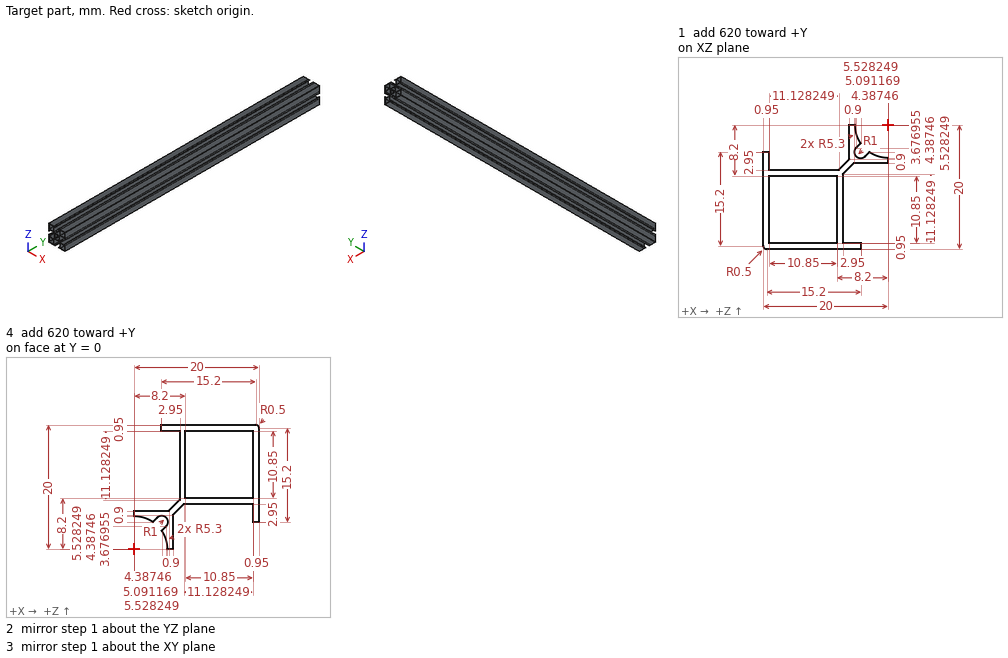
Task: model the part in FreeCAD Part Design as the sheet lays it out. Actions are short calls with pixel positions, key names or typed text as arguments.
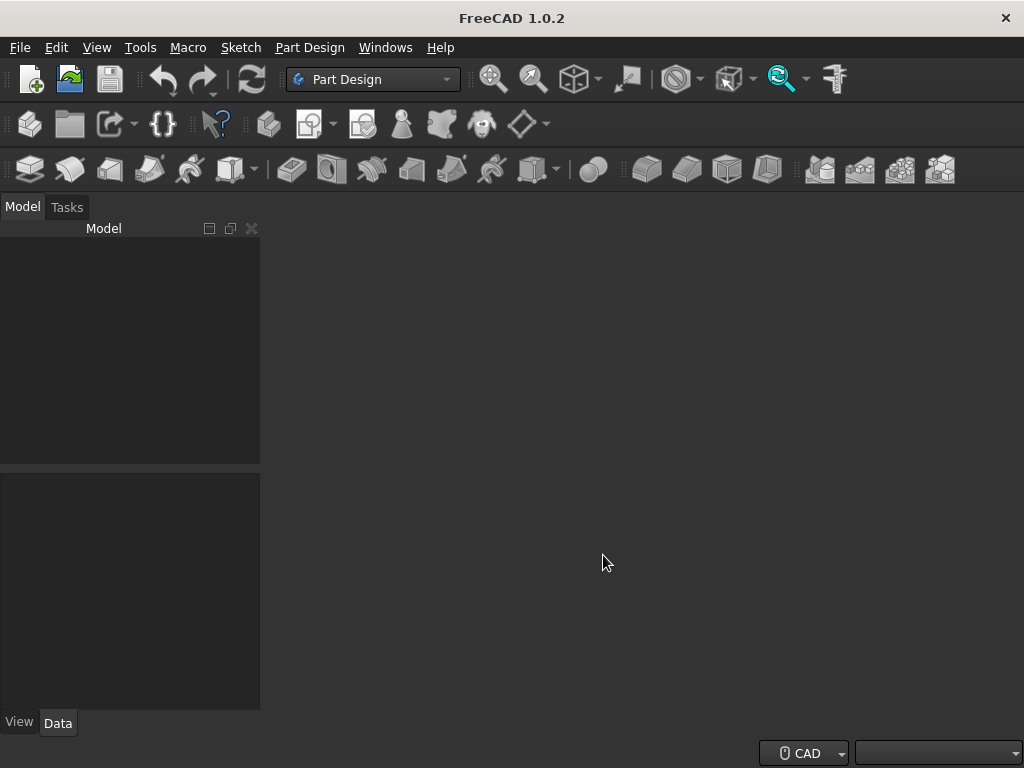
click(30, 80)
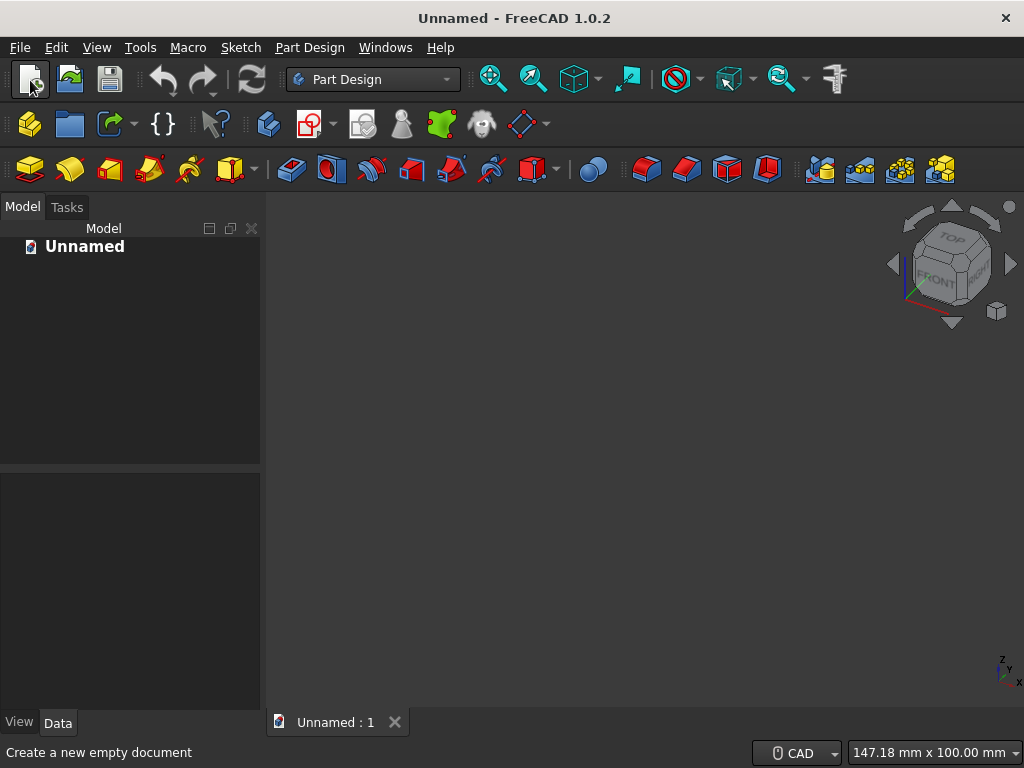
click(310, 124)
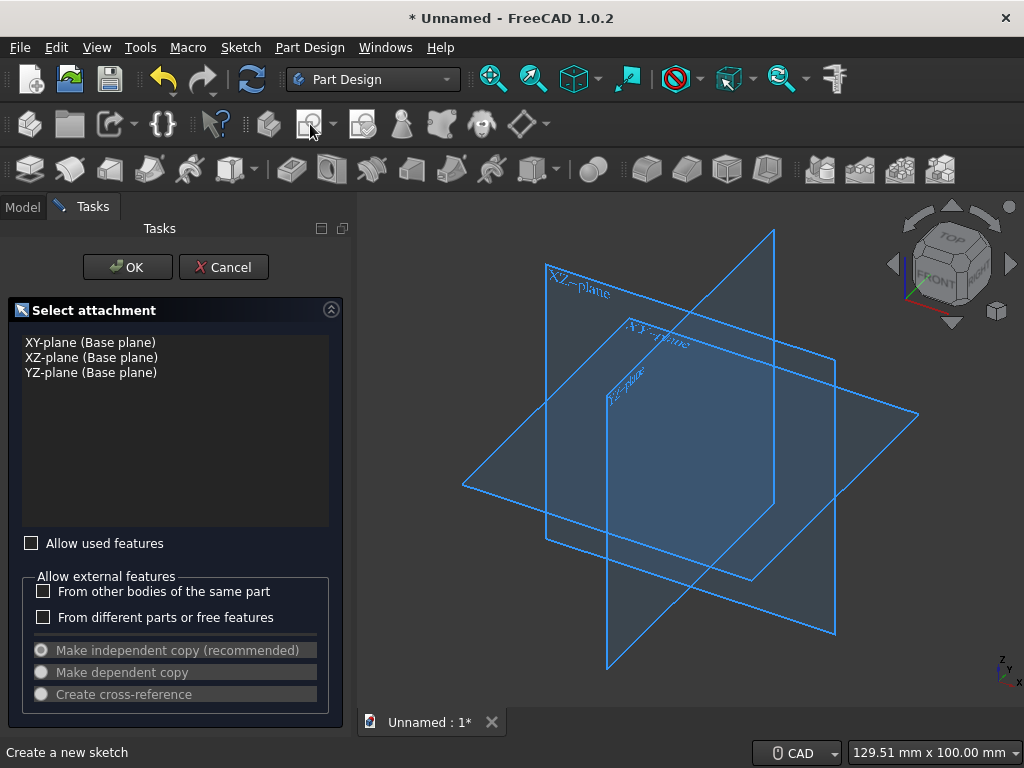
click(82, 358)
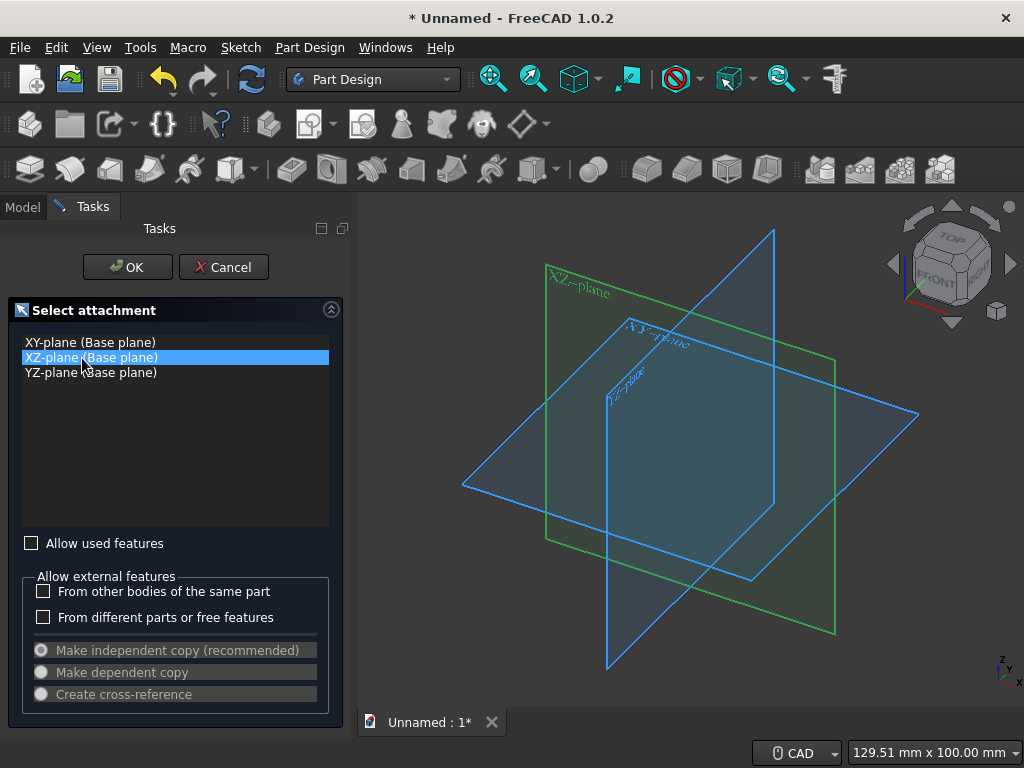
click(128, 267)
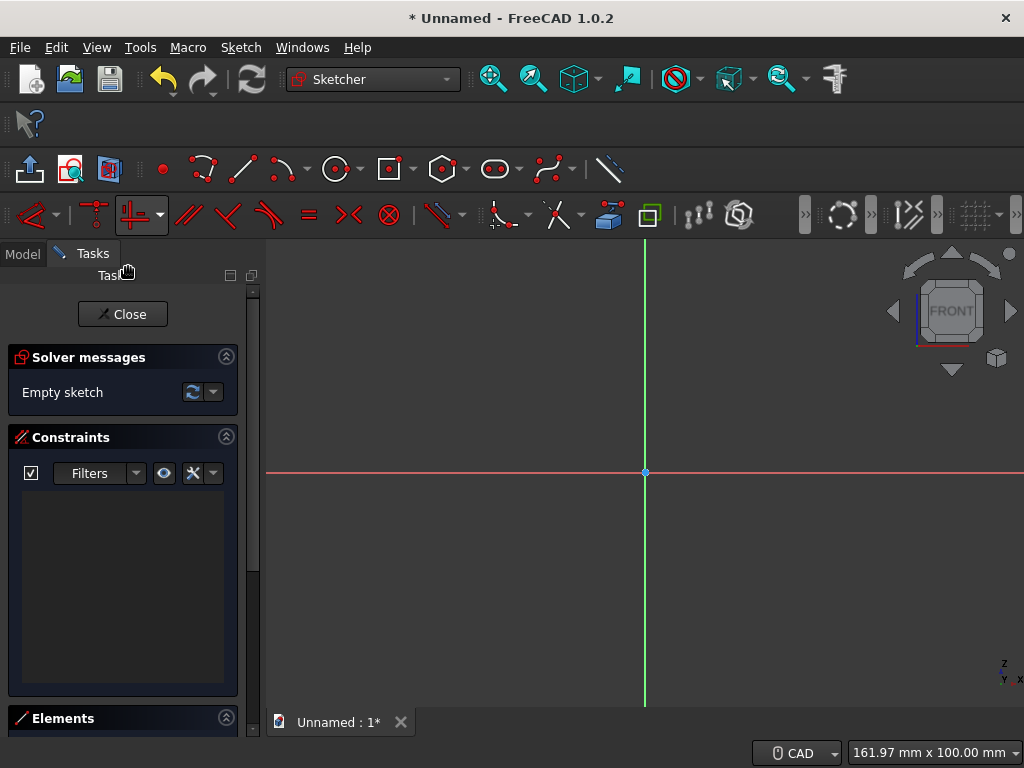
scroll(608, 540, up, 6)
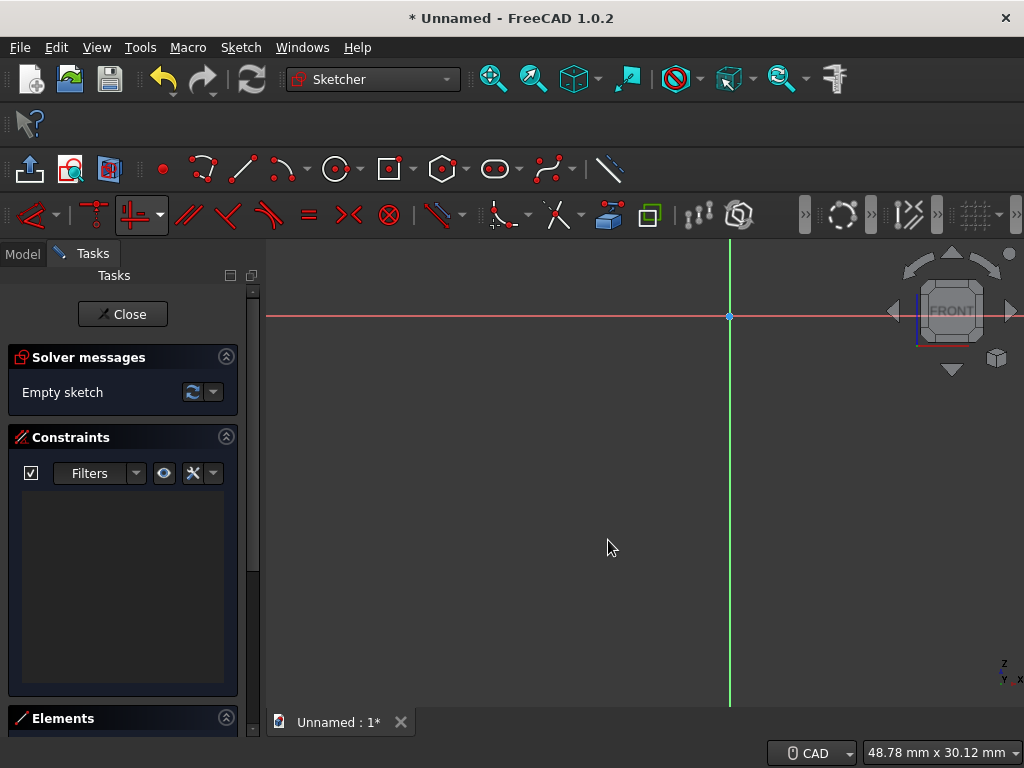
click(204, 170)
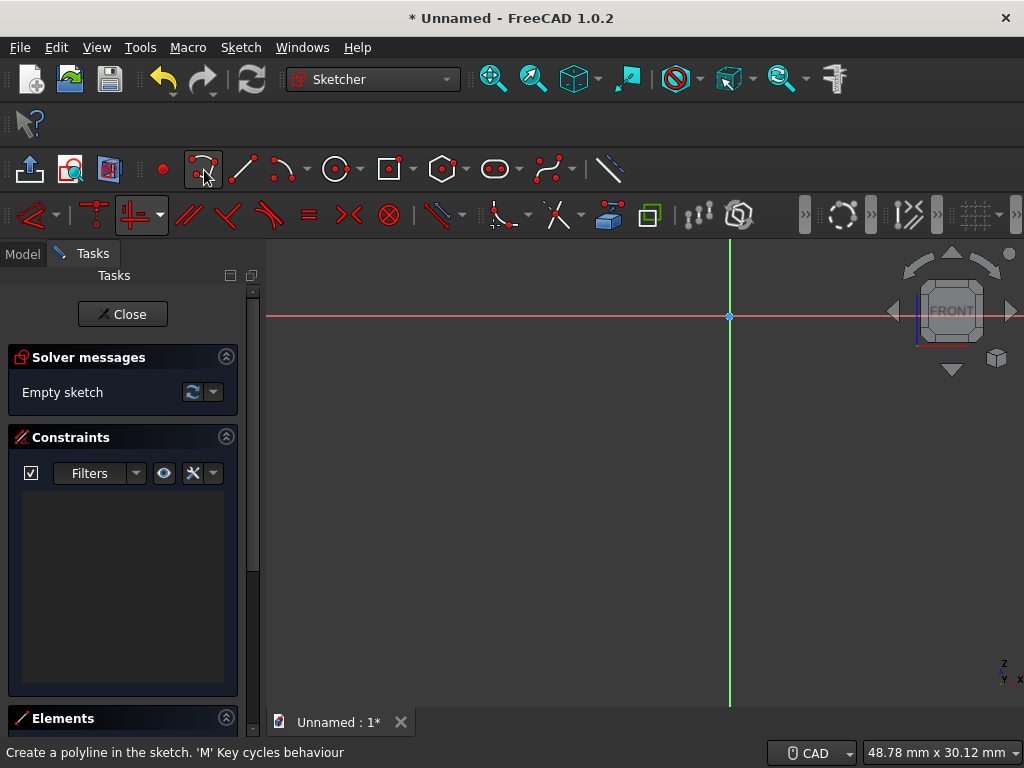
click(419, 619)
click(419, 383)
click(434, 383)
click(434, 429)
click(607, 429)
click(633, 402)
click(633, 316)
click(647, 325)
right_click(647, 325)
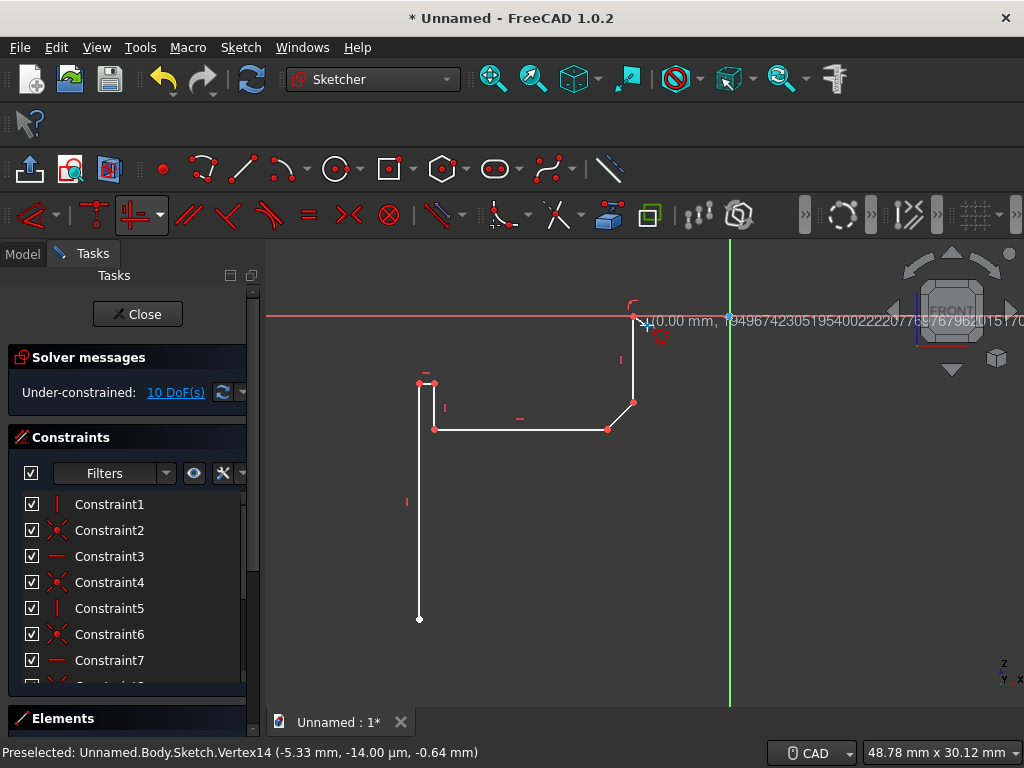
click(244, 170)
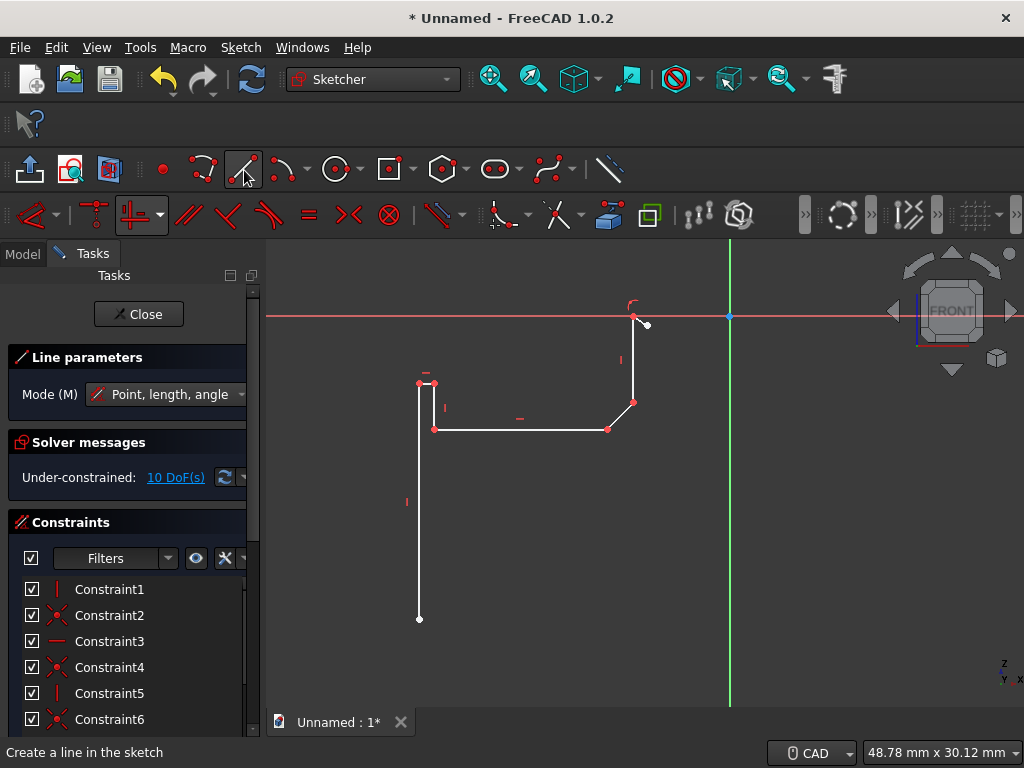
click(662, 362)
click(651, 373)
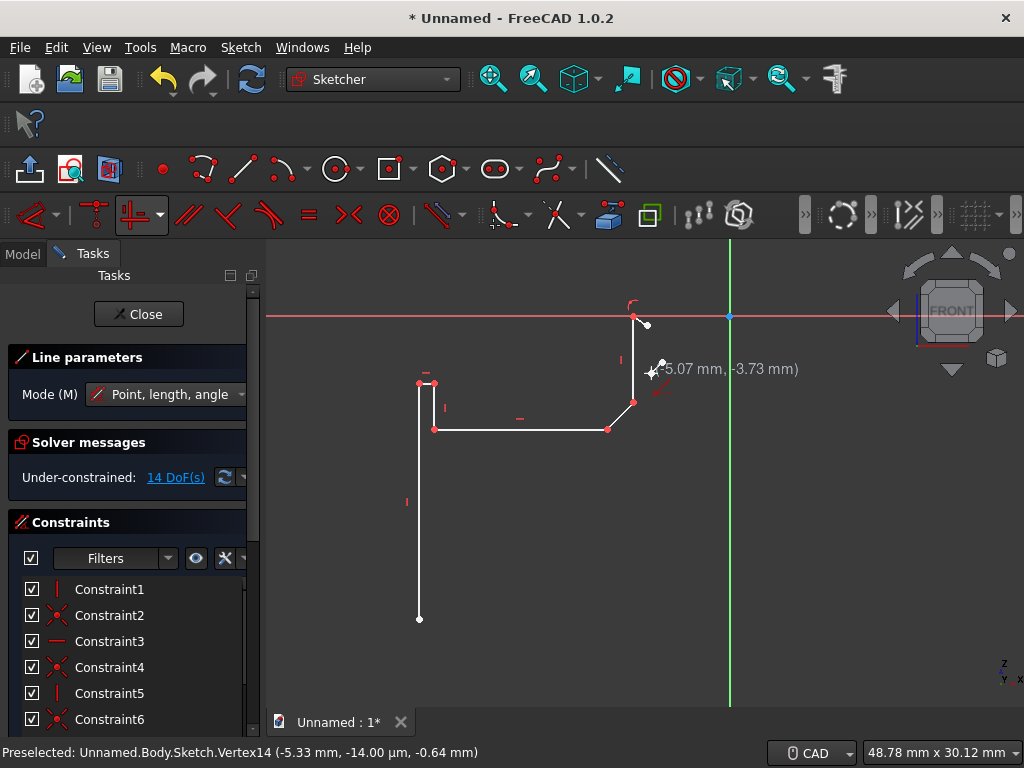
click(673, 395)
click(684, 384)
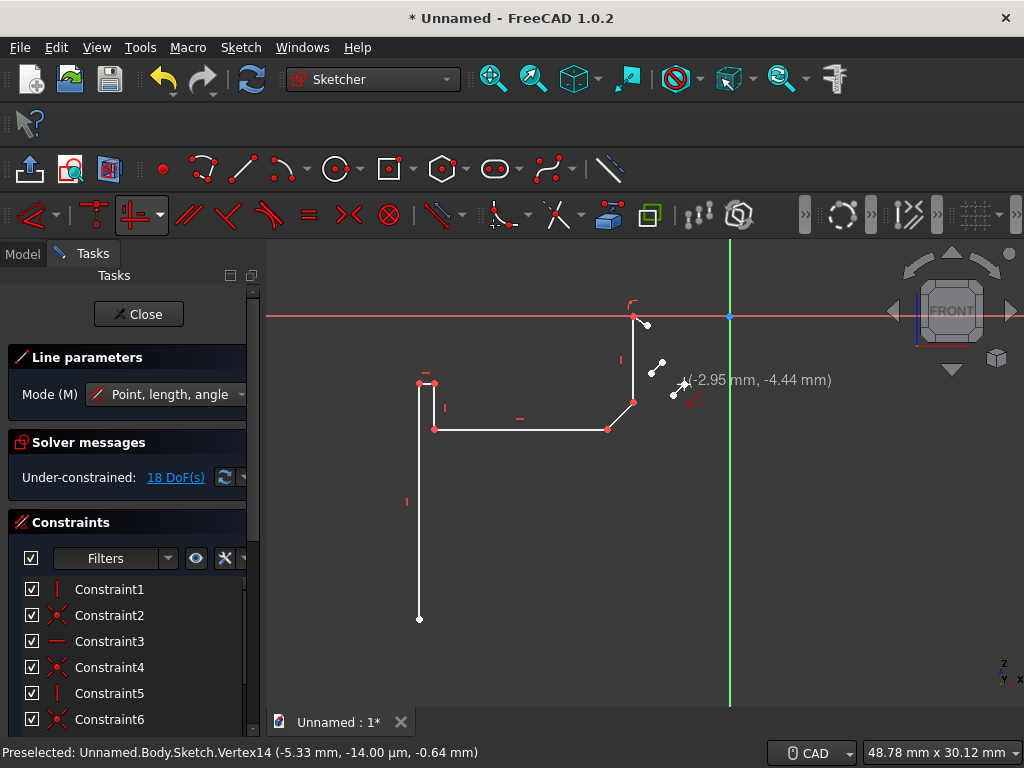
click(204, 170)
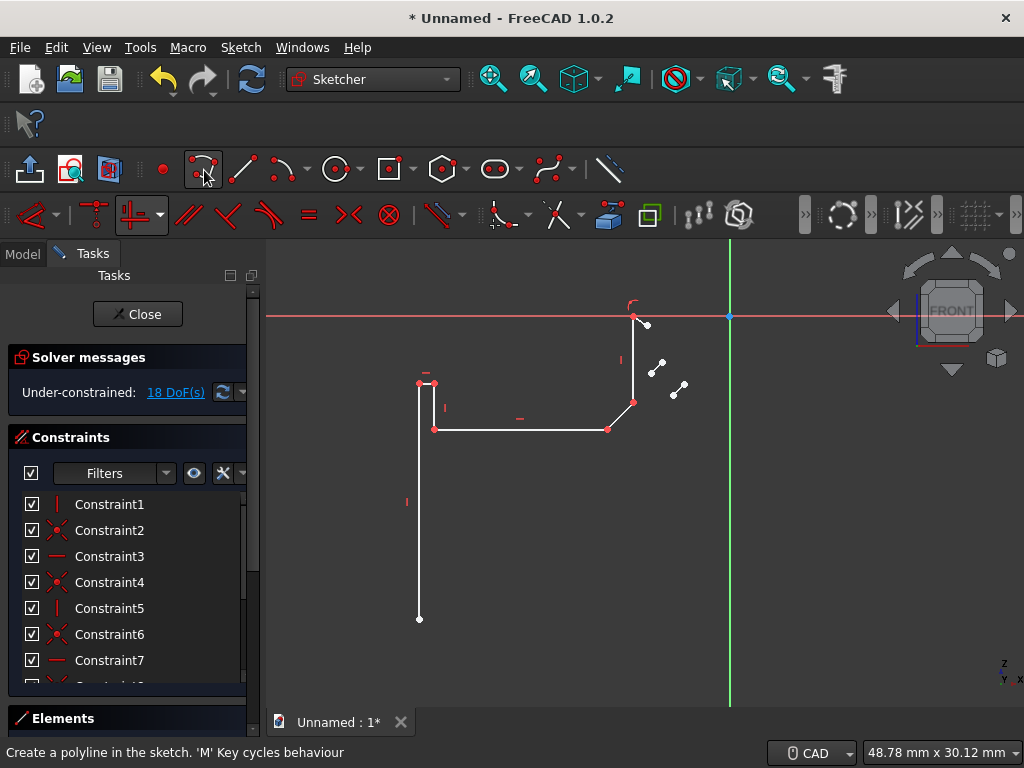
click(730, 398)
click(721, 412)
click(644, 412)
click(617, 439)
click(617, 612)
click(663, 612)
click(663, 627)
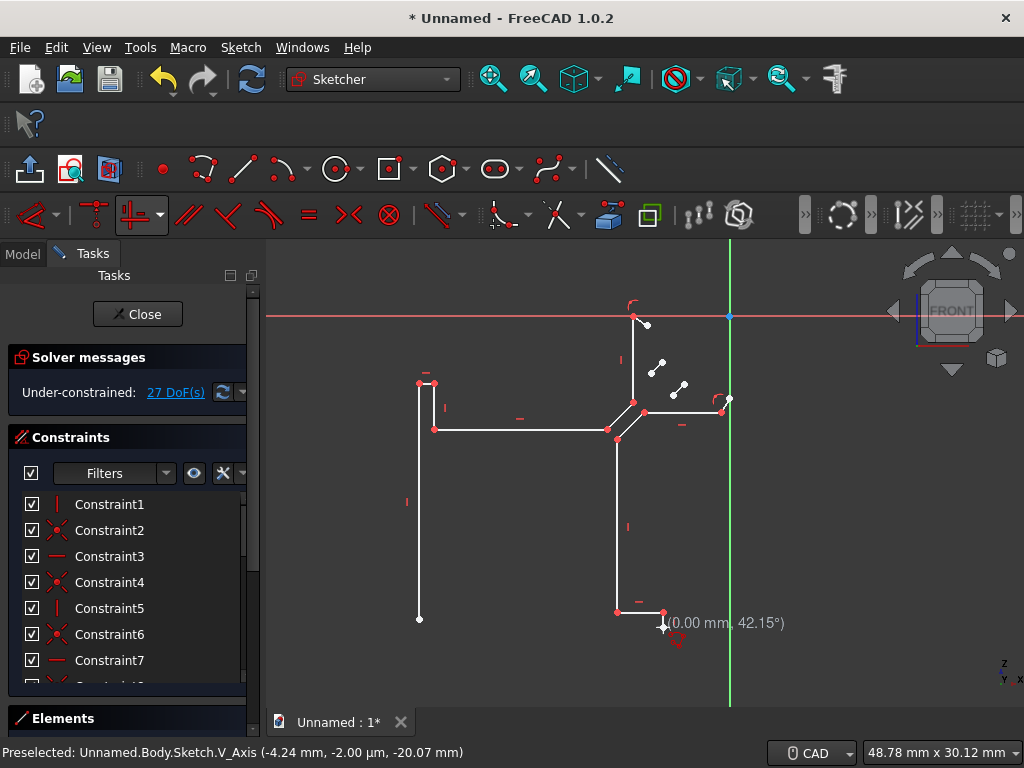
scroll(427, 627, up, 2)